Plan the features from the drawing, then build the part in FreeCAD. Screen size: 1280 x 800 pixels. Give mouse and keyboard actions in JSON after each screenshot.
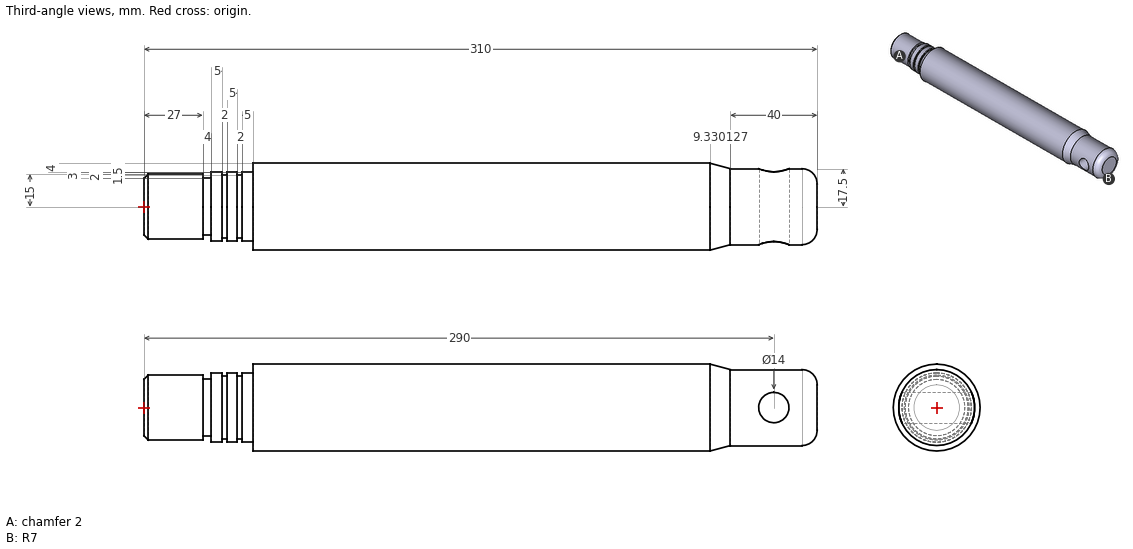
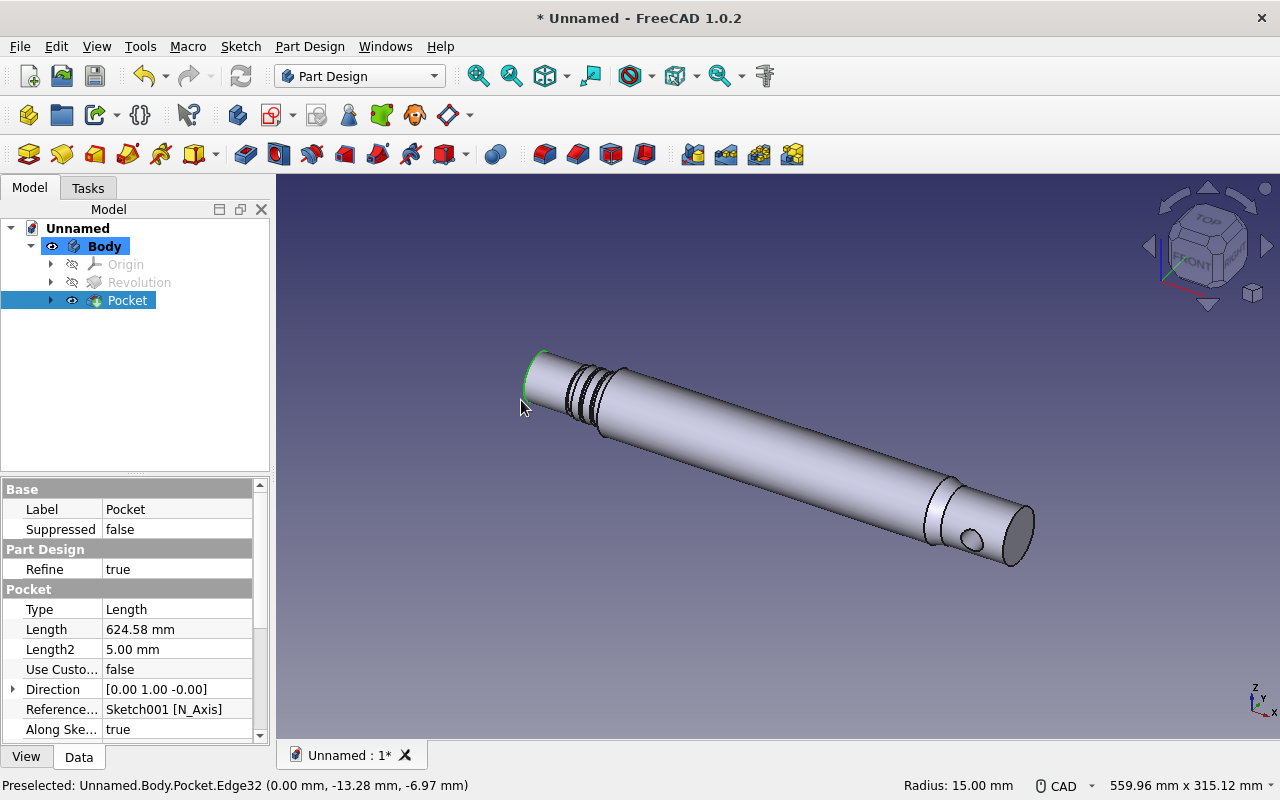
{"action": "left_click", "coordinate": [578, 154]}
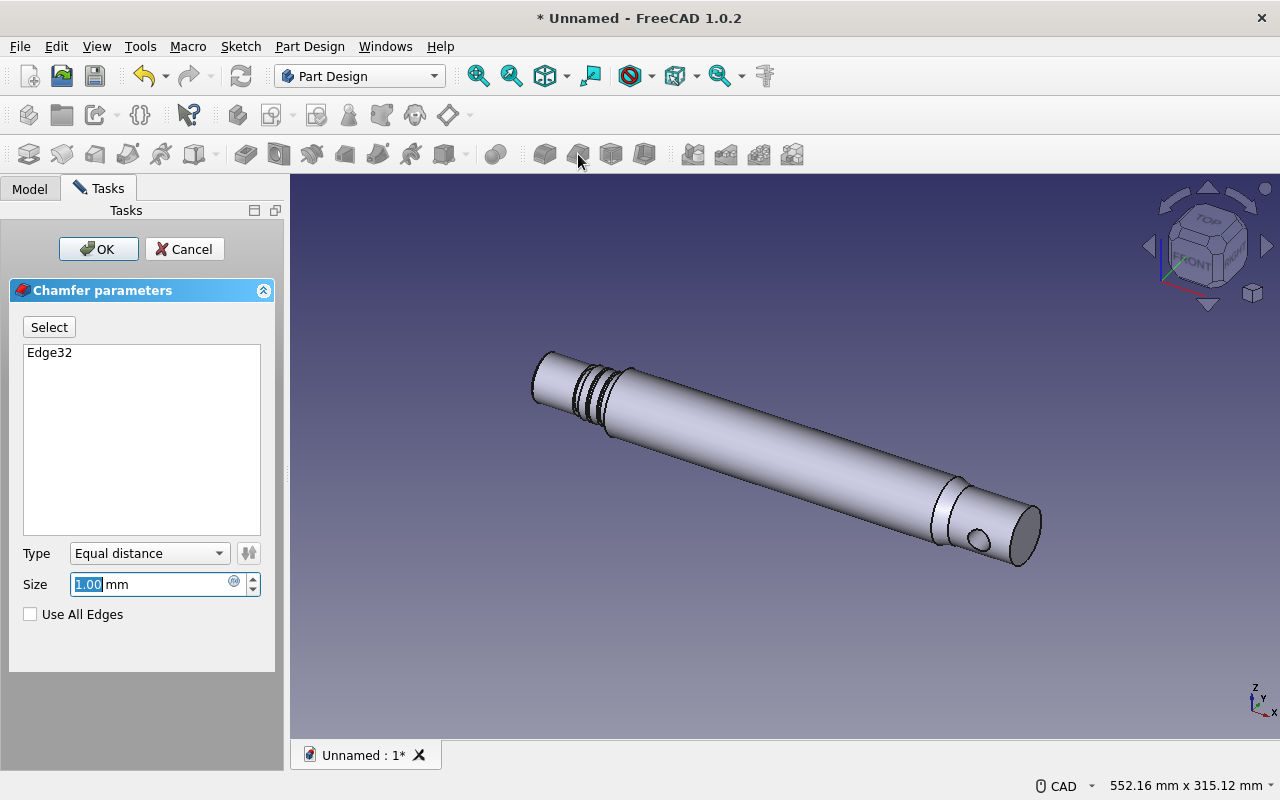
{"action": "type", "text": "2"}
{"action": "key", "text": "Tab"}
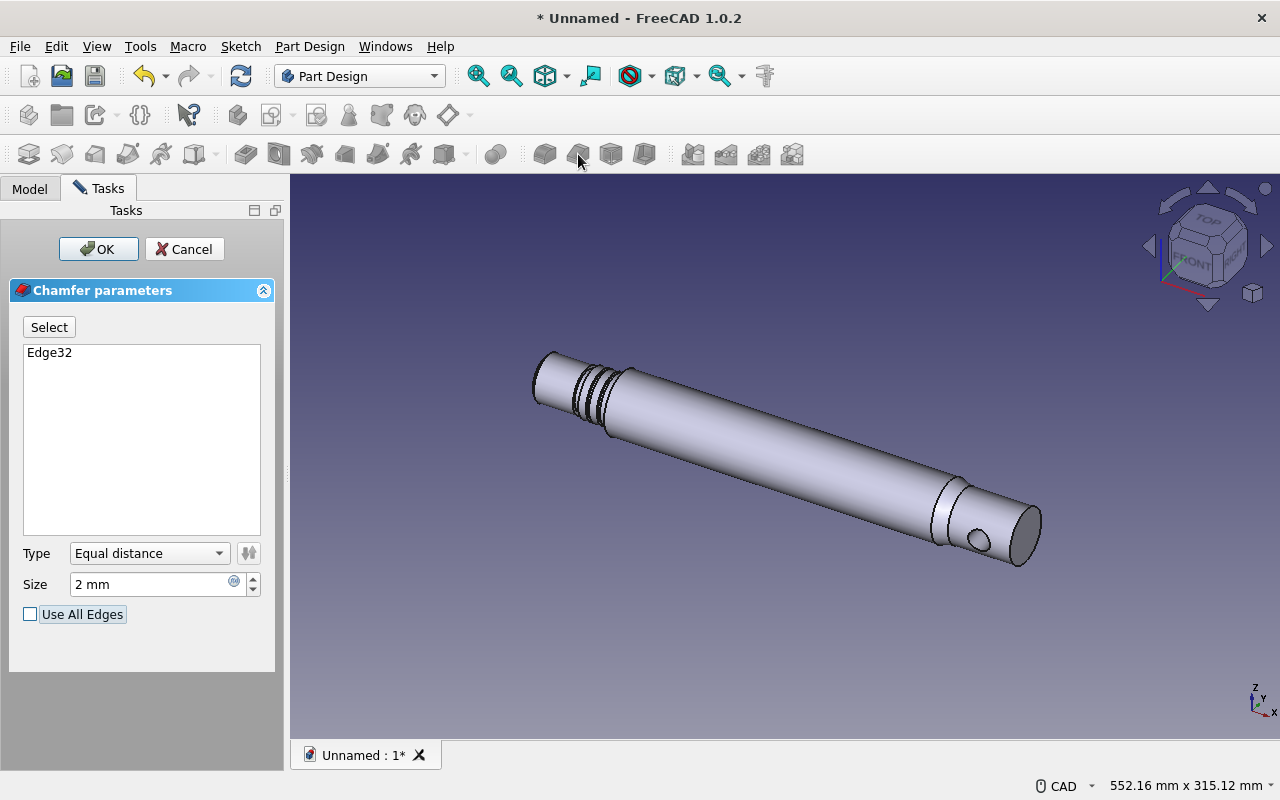
{"action": "left_click", "coordinate": [99, 249]}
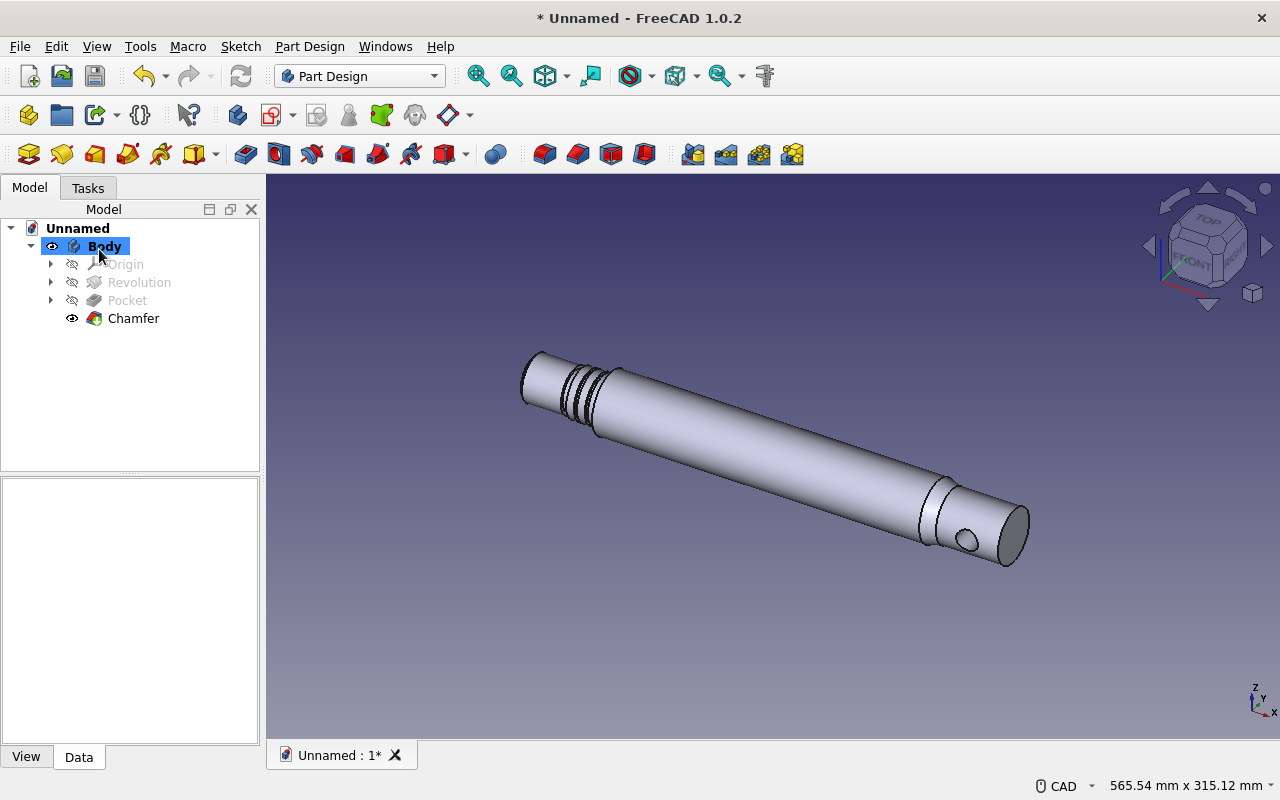
{"action": "left_click", "coordinate": [998, 551]}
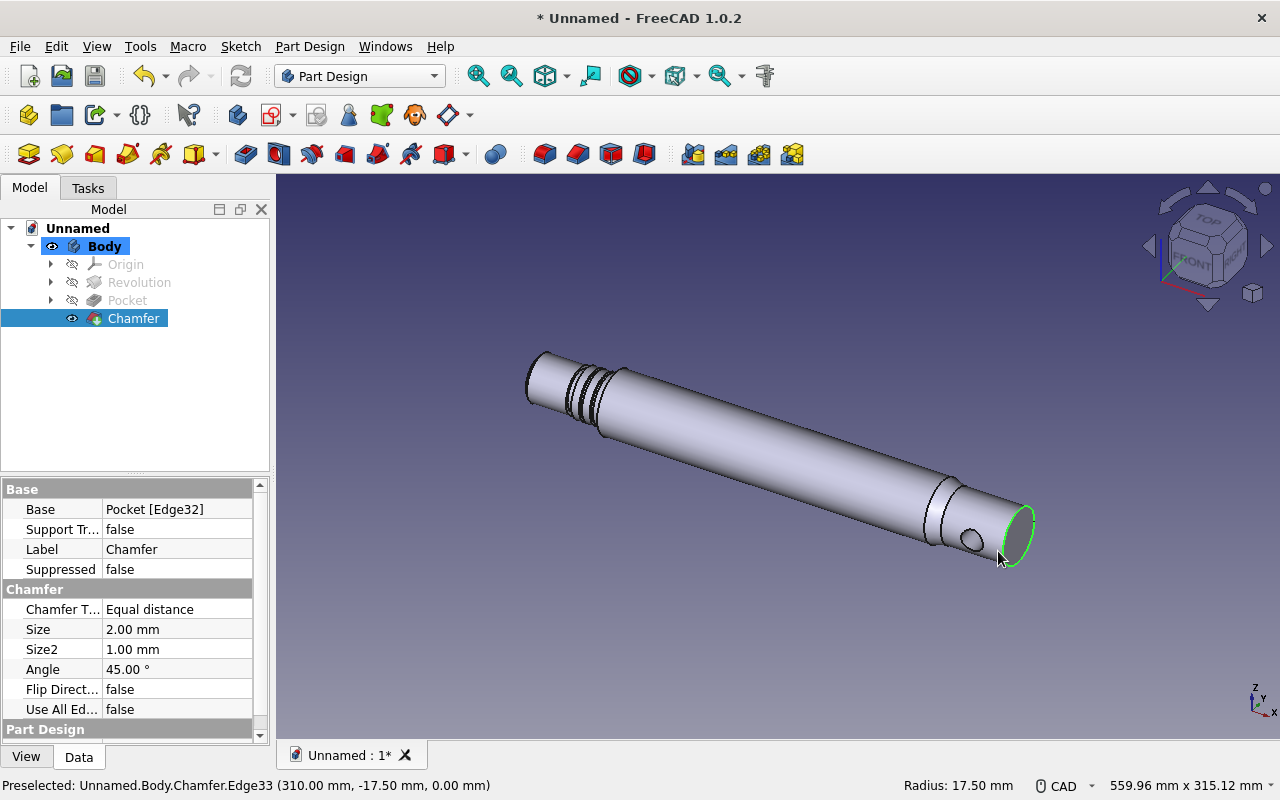
{"action": "left_click", "coordinate": [545, 154]}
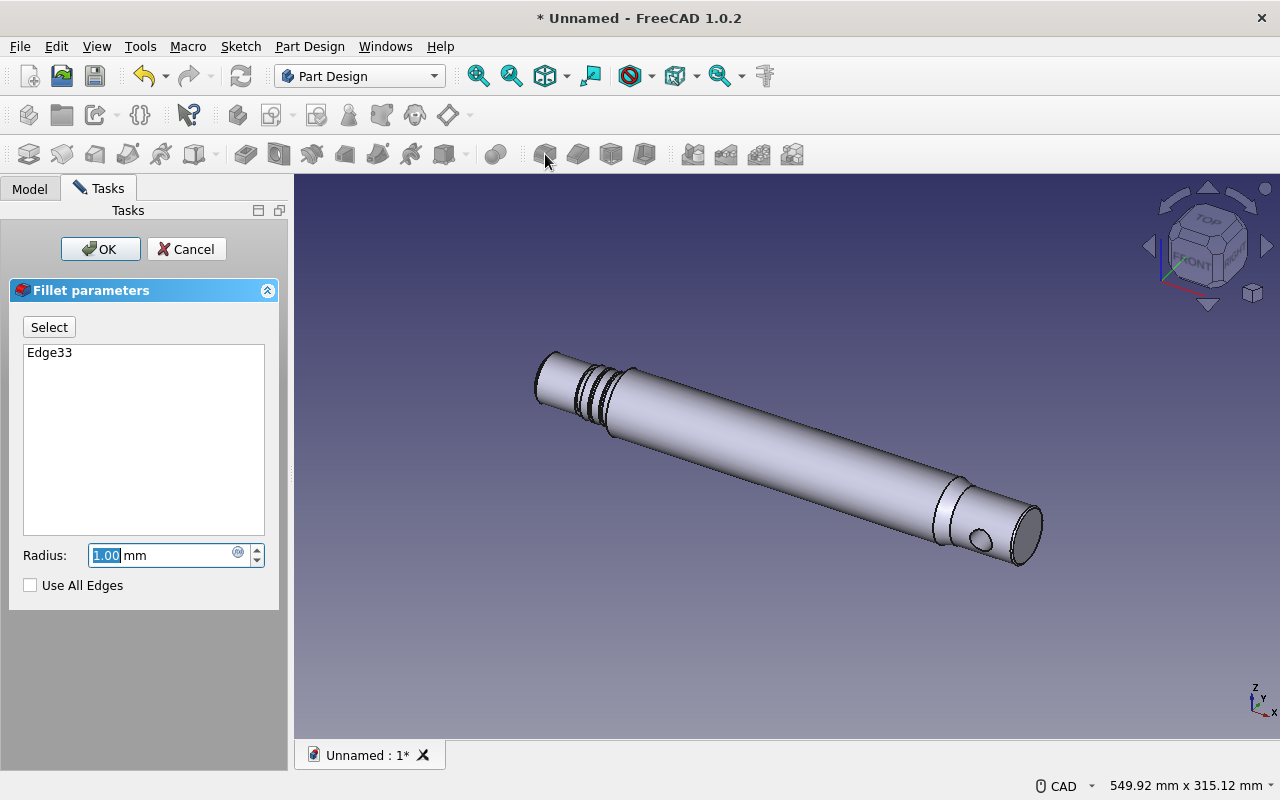
{"action": "type", "text": "7"}
{"action": "key", "text": "Tab"}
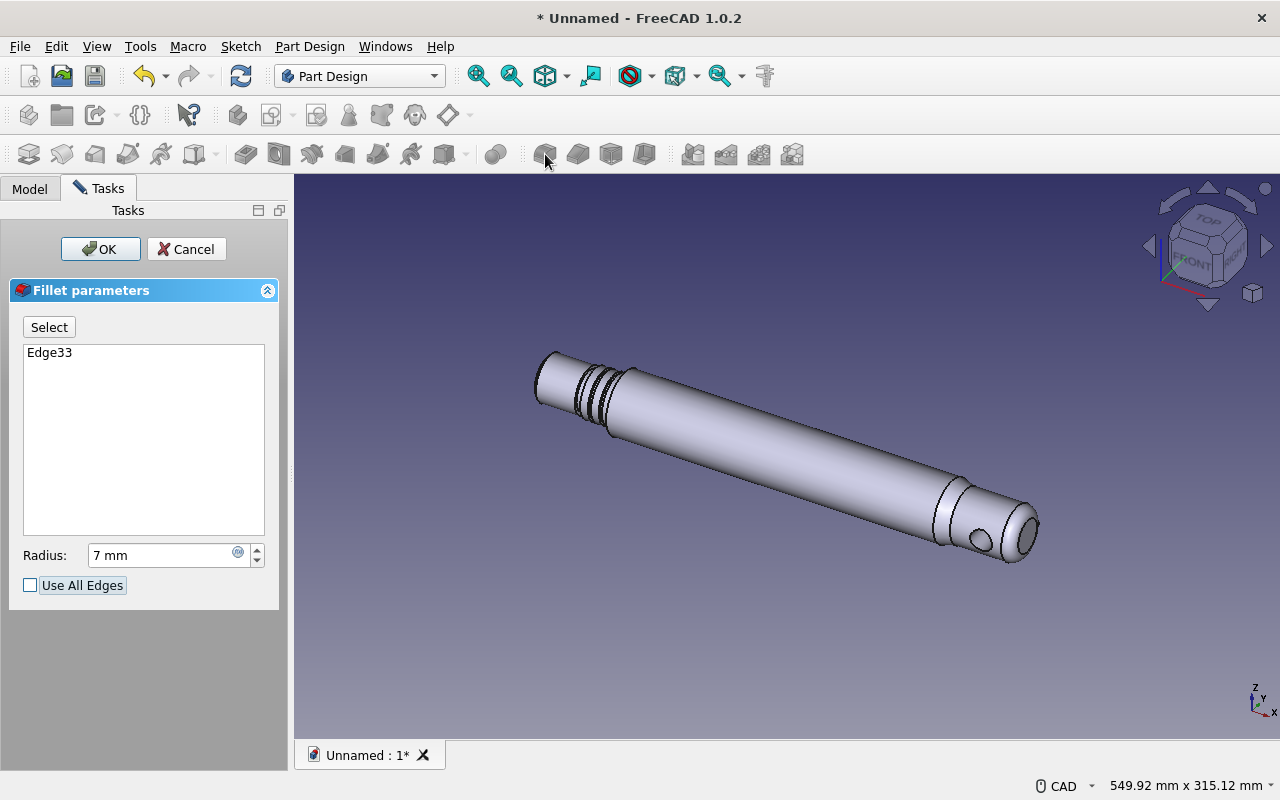
{"action": "left_click", "coordinate": [101, 249]}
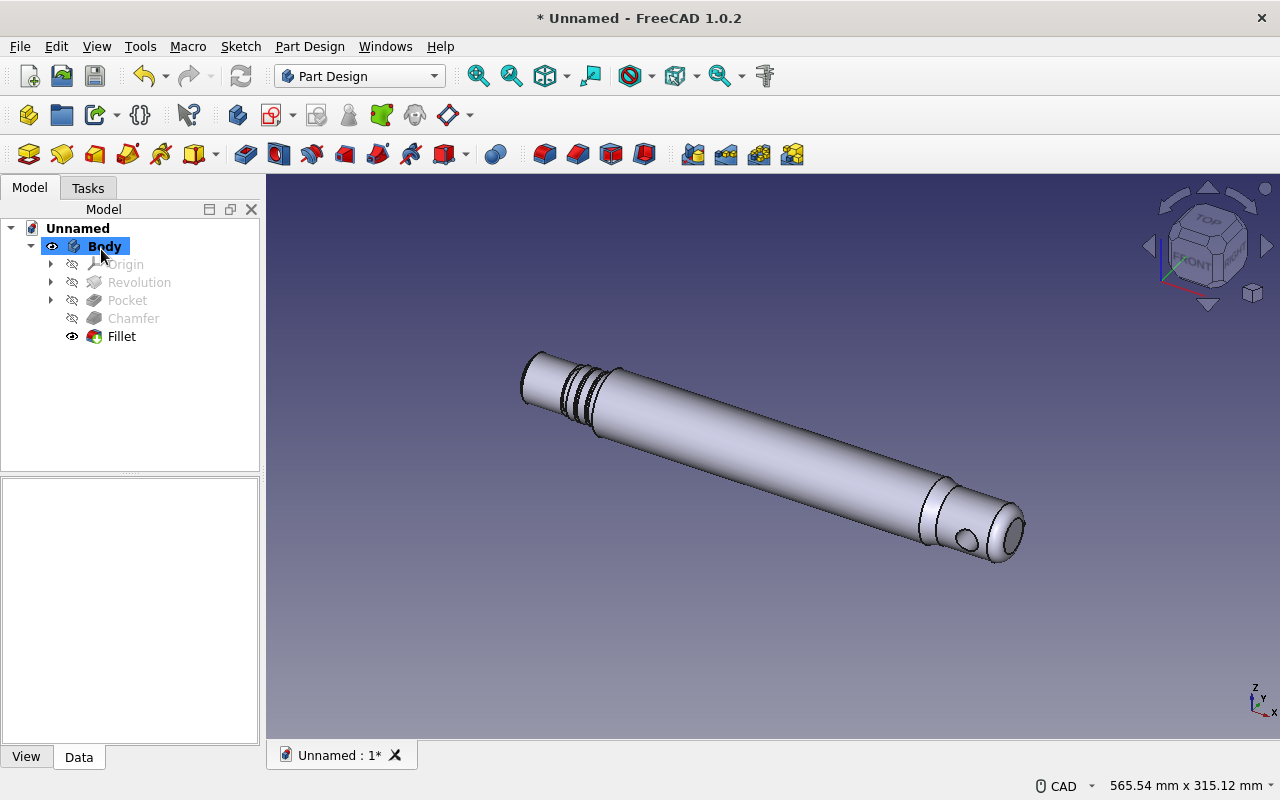
{"action": "key", "text": "0"}